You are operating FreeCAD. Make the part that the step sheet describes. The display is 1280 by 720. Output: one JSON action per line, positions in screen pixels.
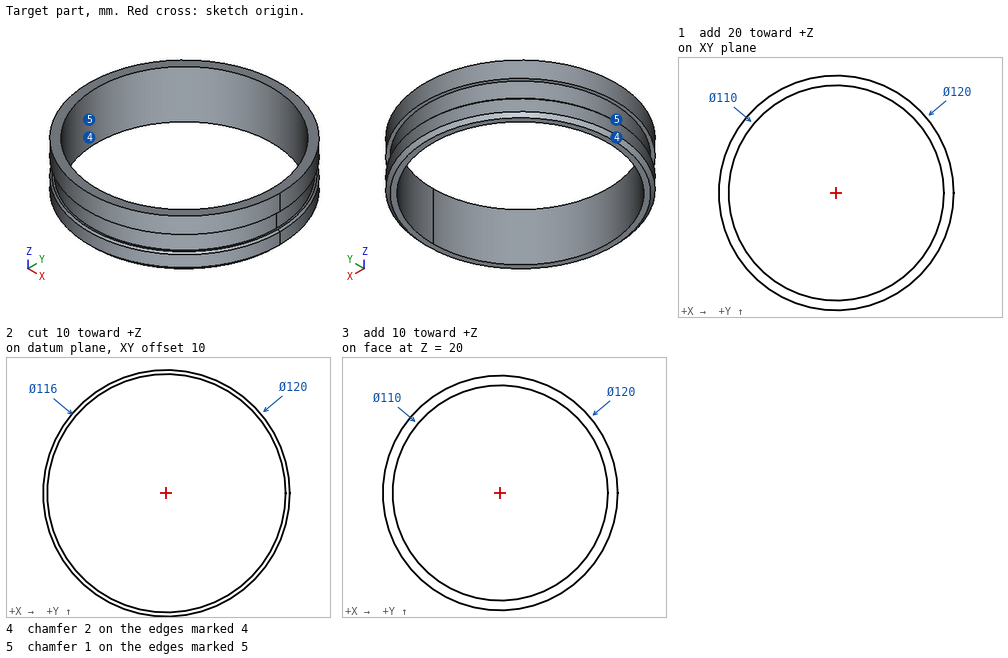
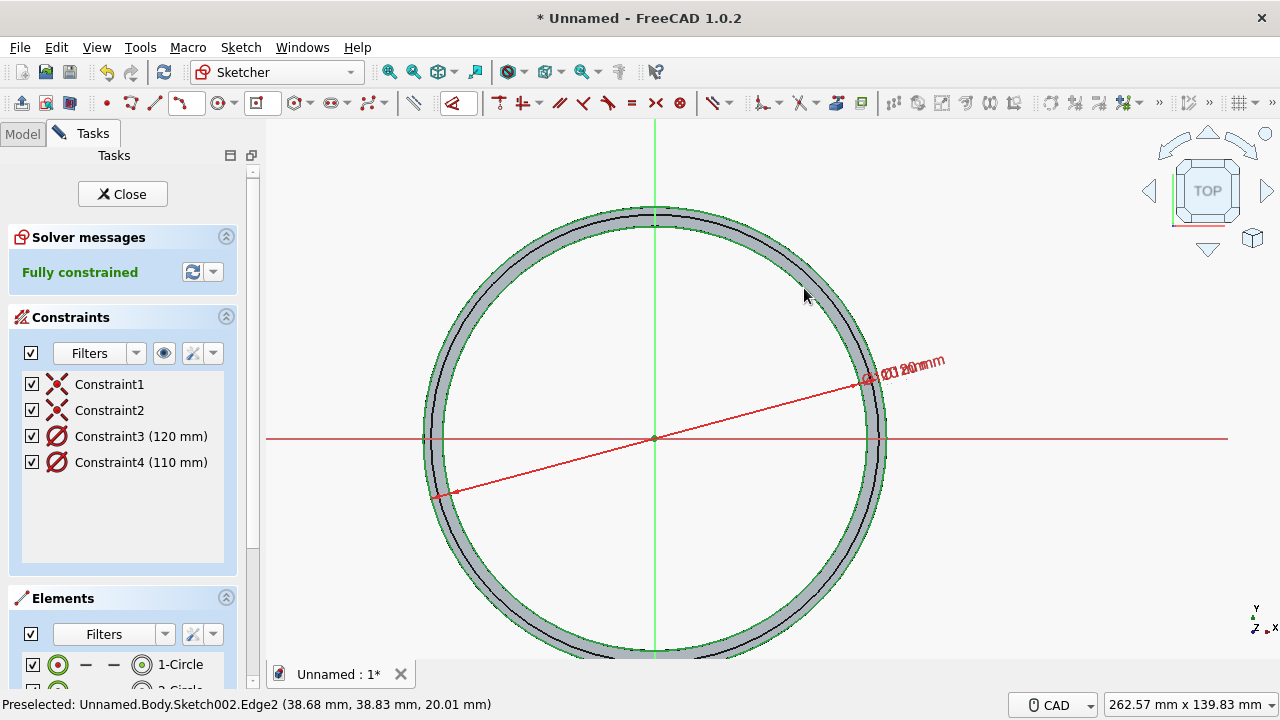
{"action": "left_click", "coordinate": [123, 194]}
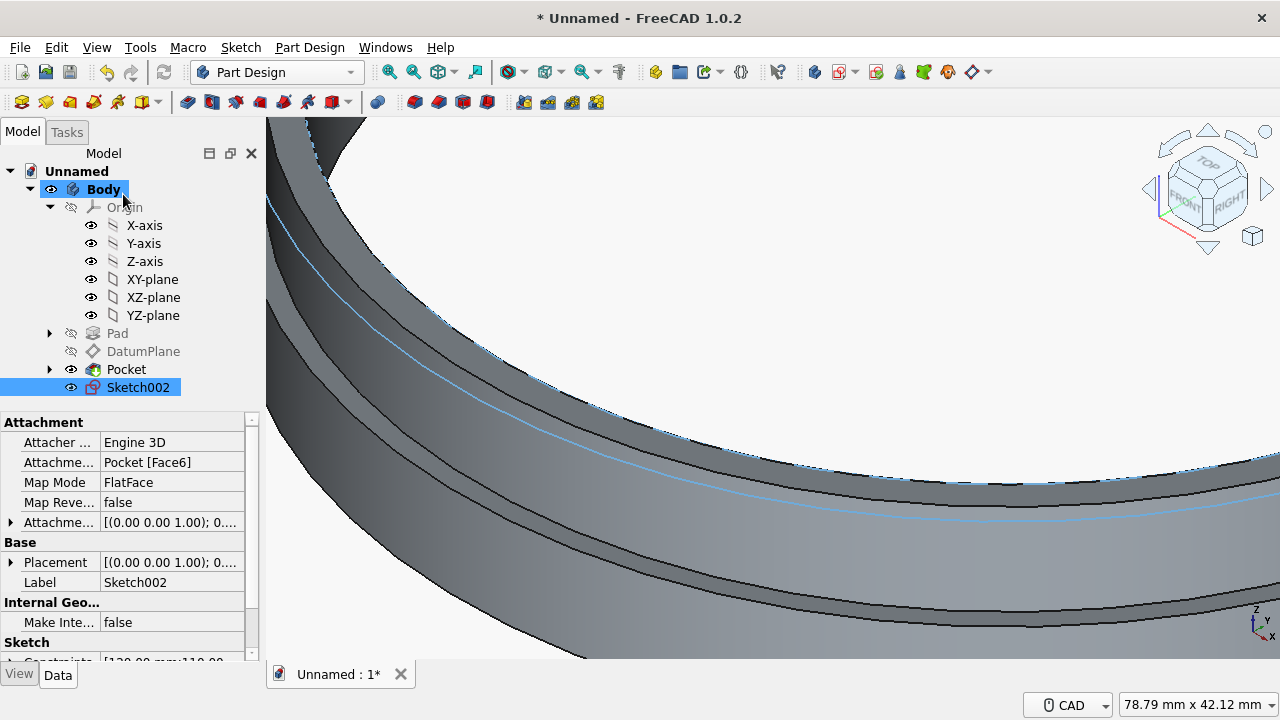
{"action": "left_click", "coordinate": [22, 102]}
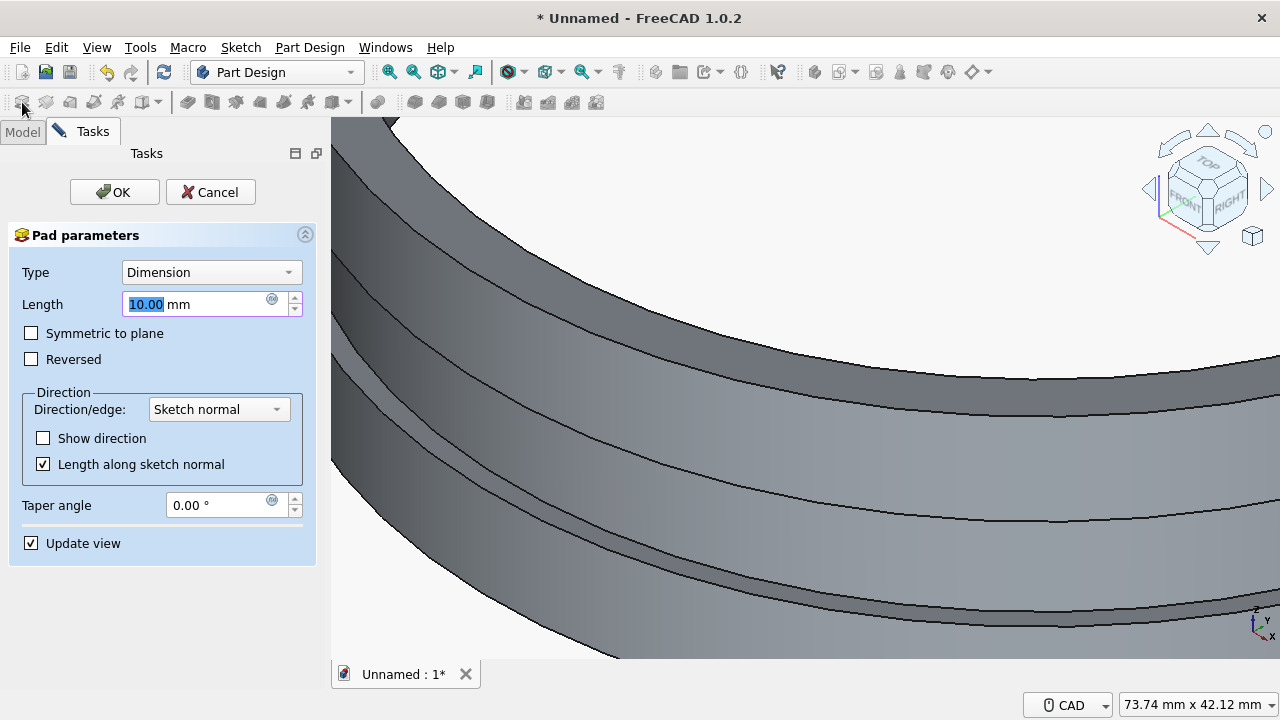
{"action": "type", "text": "10"}
{"action": "key", "text": "Tab"}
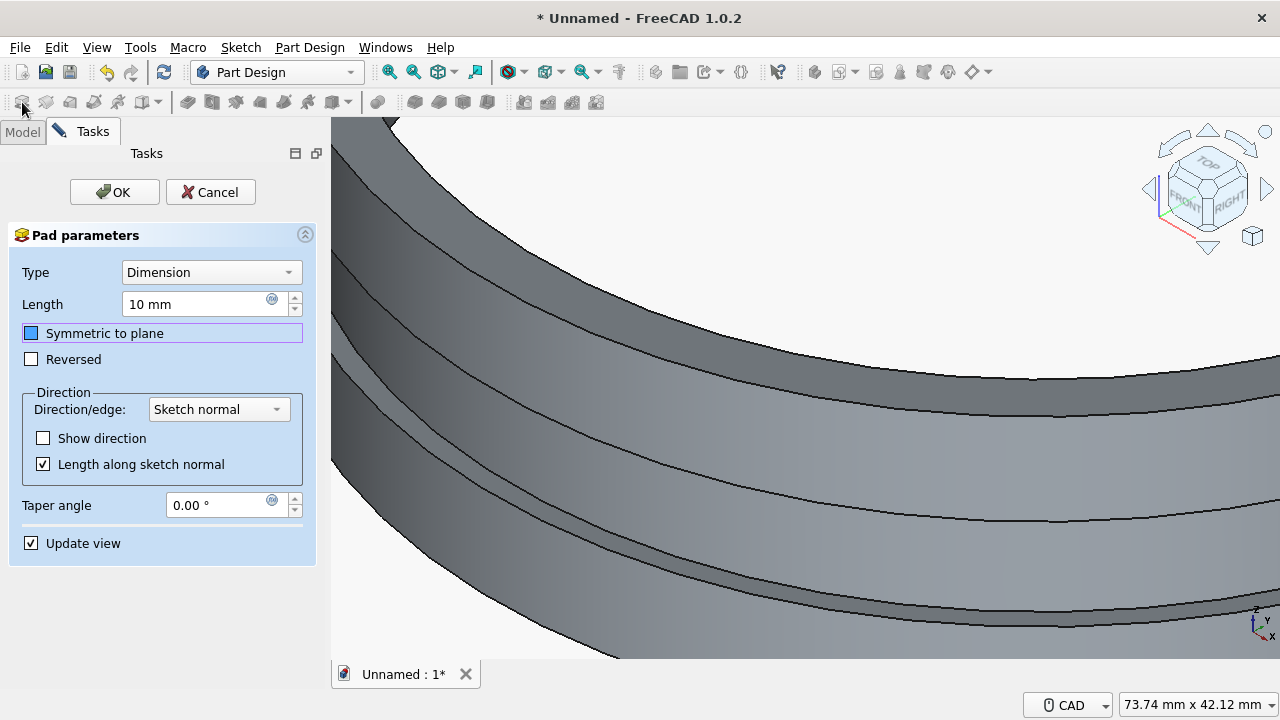
{"action": "left_click", "coordinate": [115, 192]}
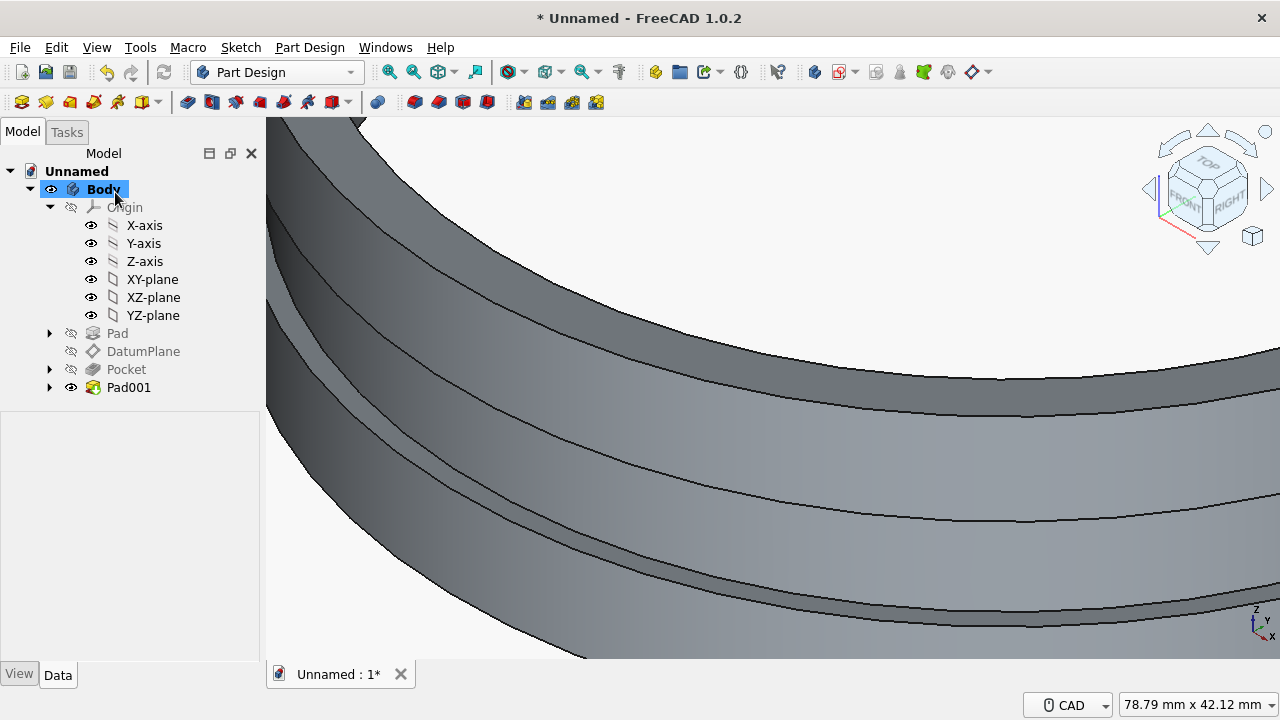
{"action": "key", "text": "v f"}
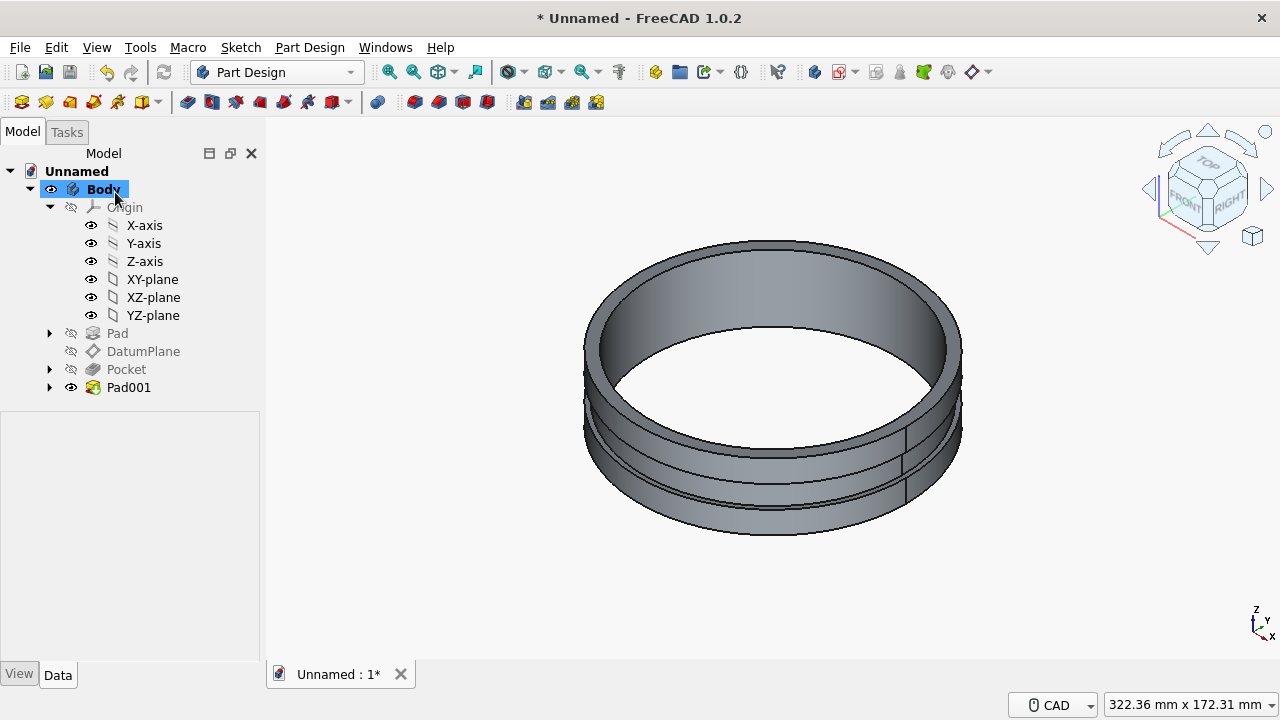
{"action": "key", "text": "2"}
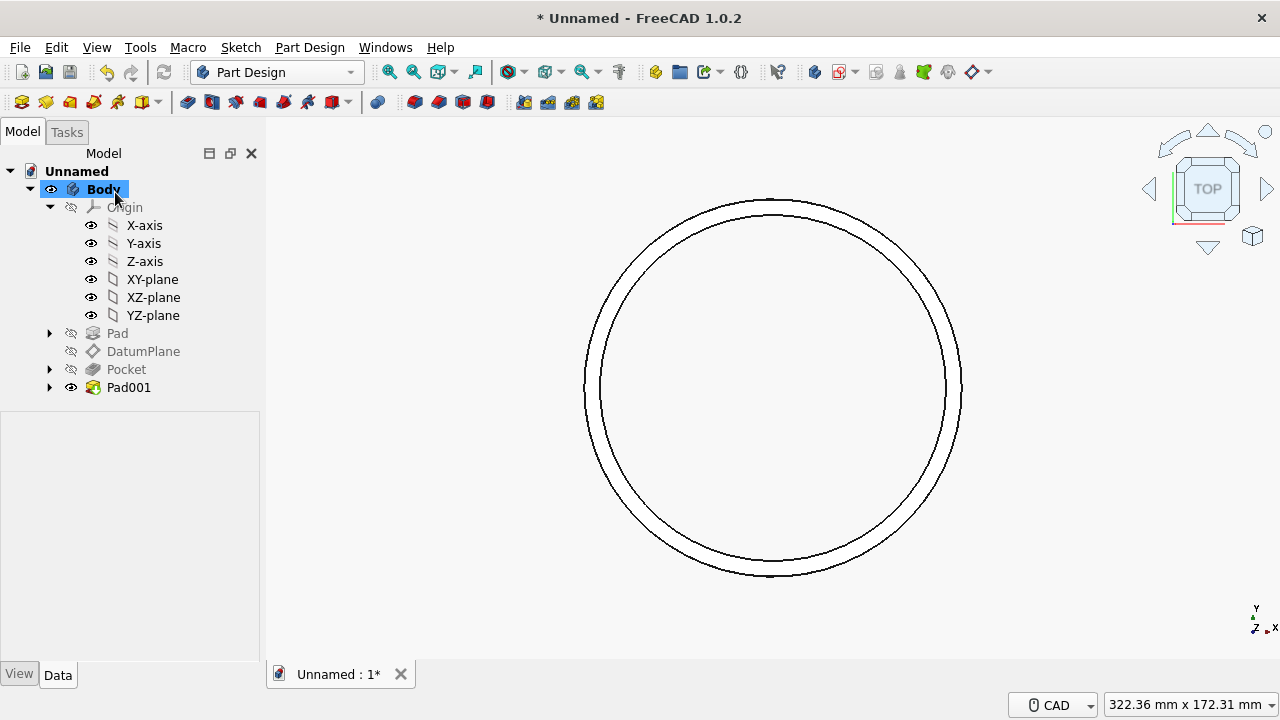
{"action": "key", "text": "0"}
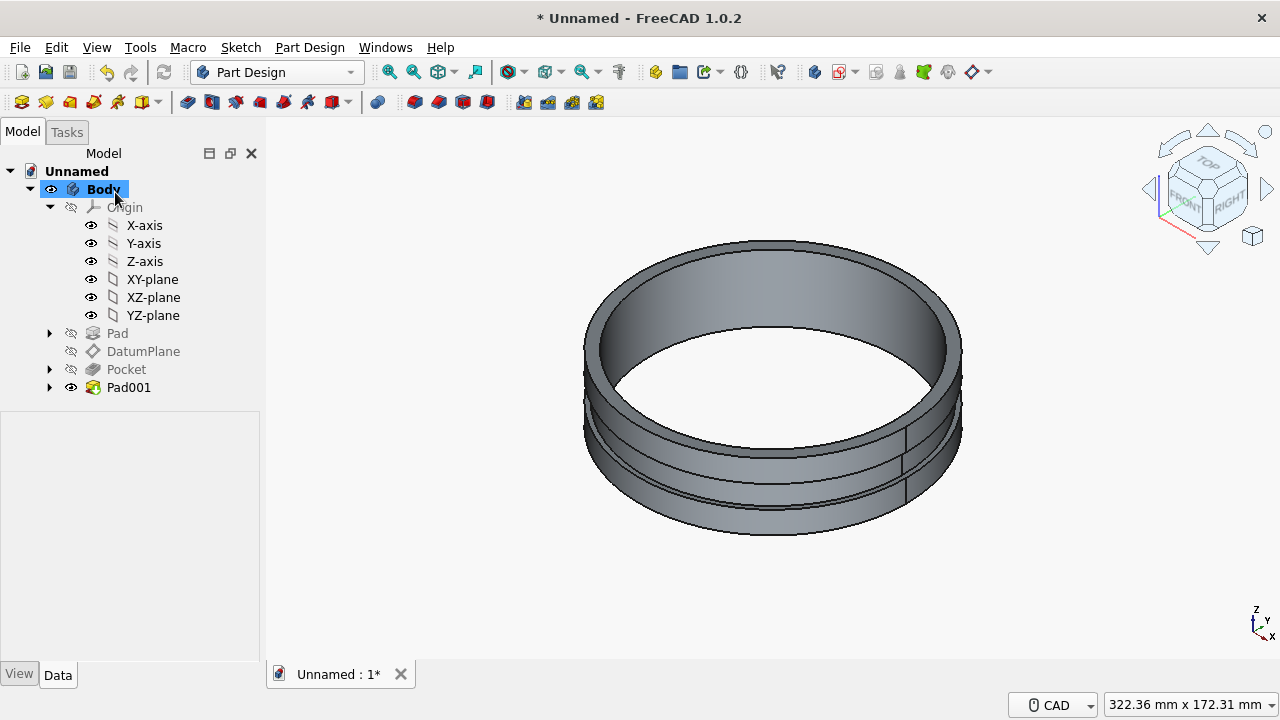
{"action": "key", "text": "1"}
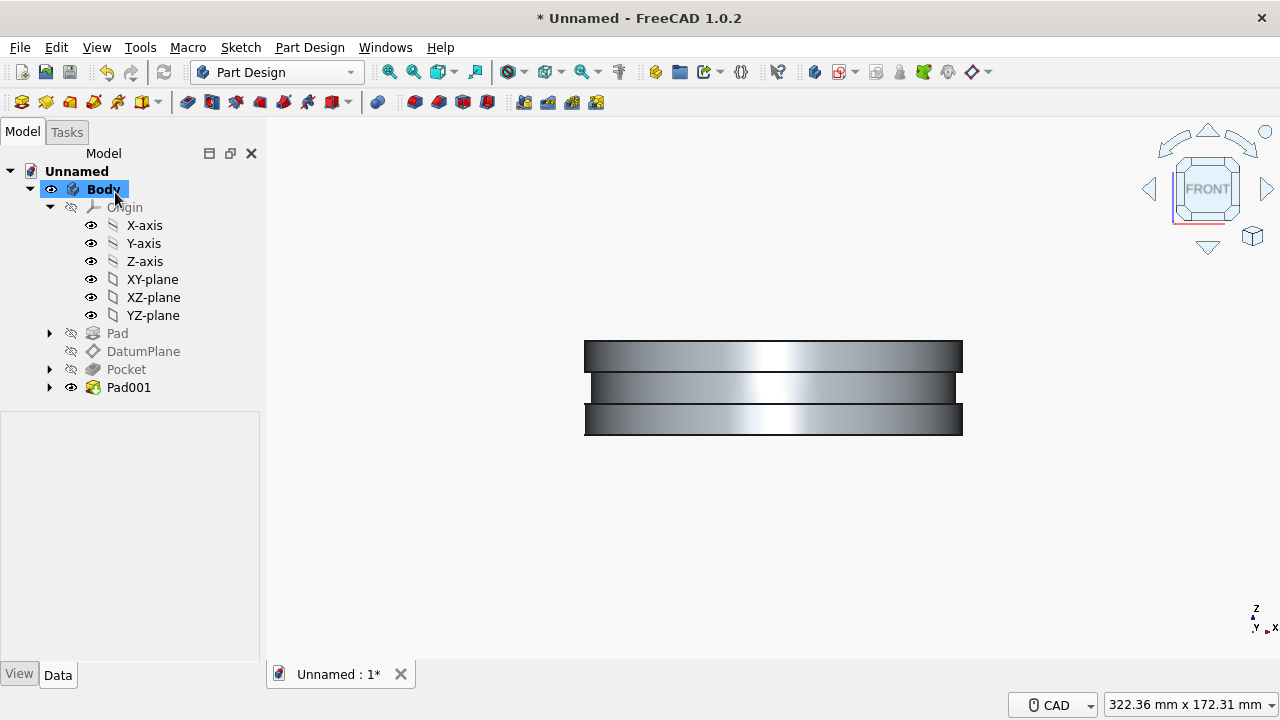
{"action": "key", "text": "v f"}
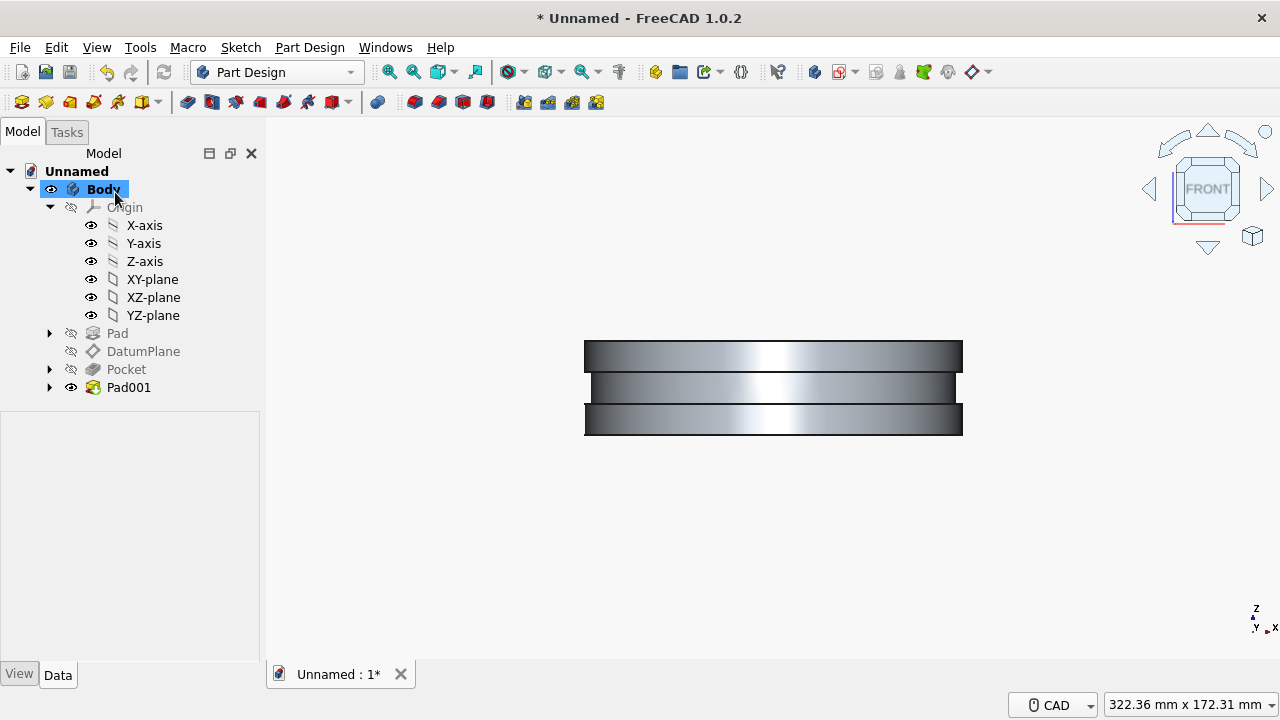
{"action": "left_click", "coordinate": [620, 434]}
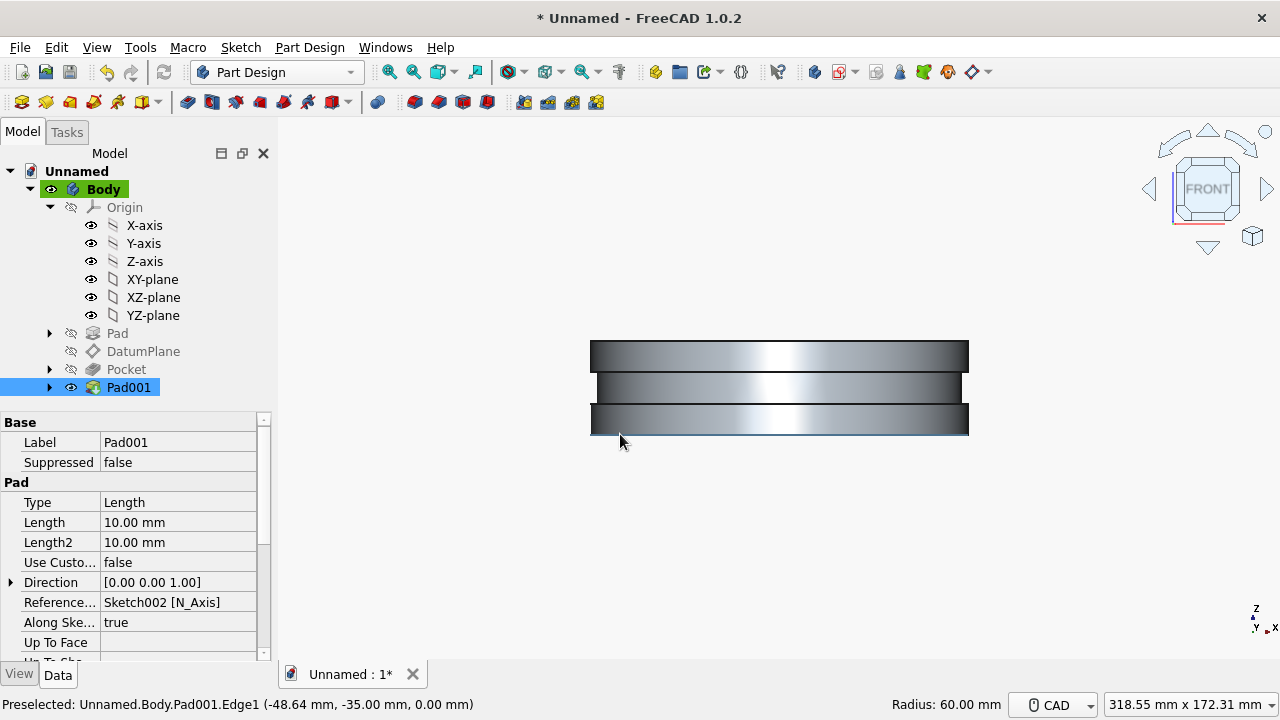
{"action": "left_click", "coordinate": [440, 102]}